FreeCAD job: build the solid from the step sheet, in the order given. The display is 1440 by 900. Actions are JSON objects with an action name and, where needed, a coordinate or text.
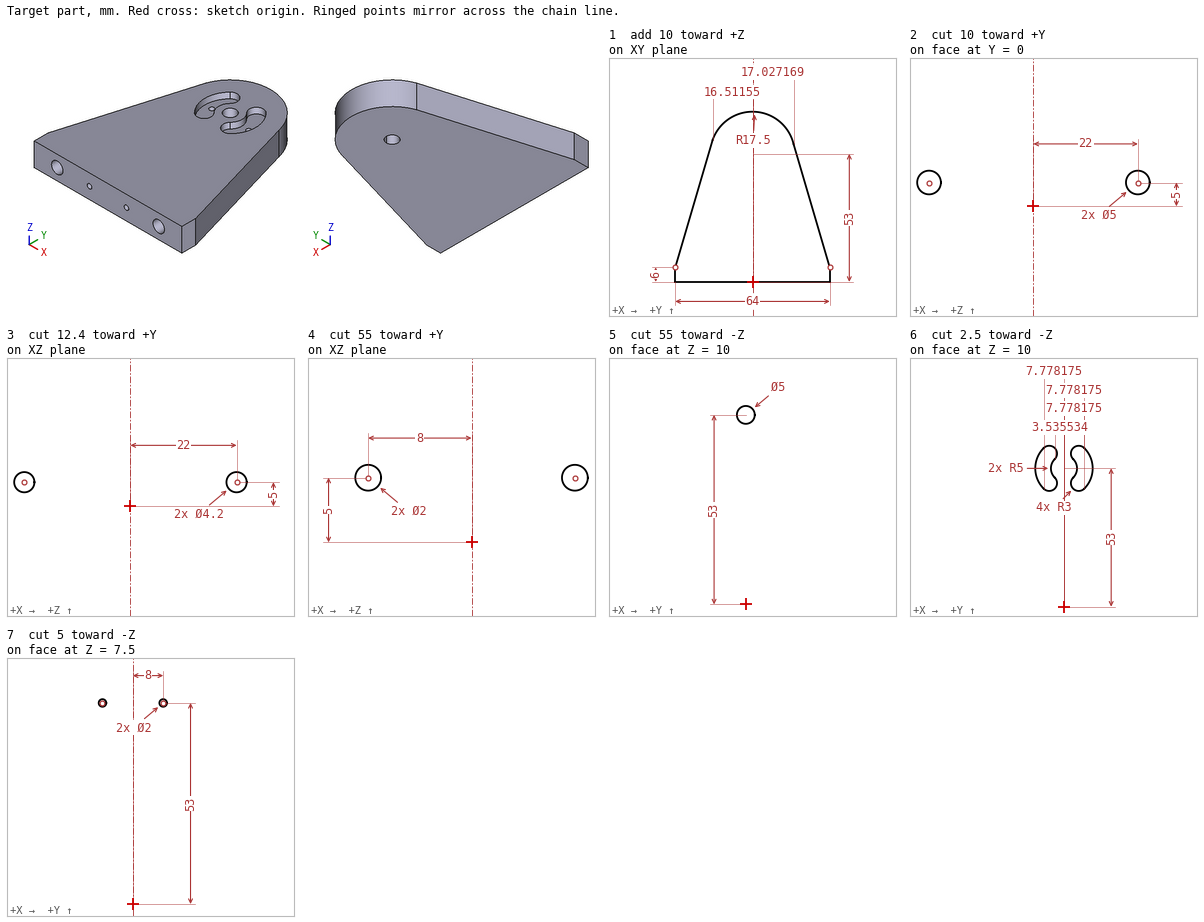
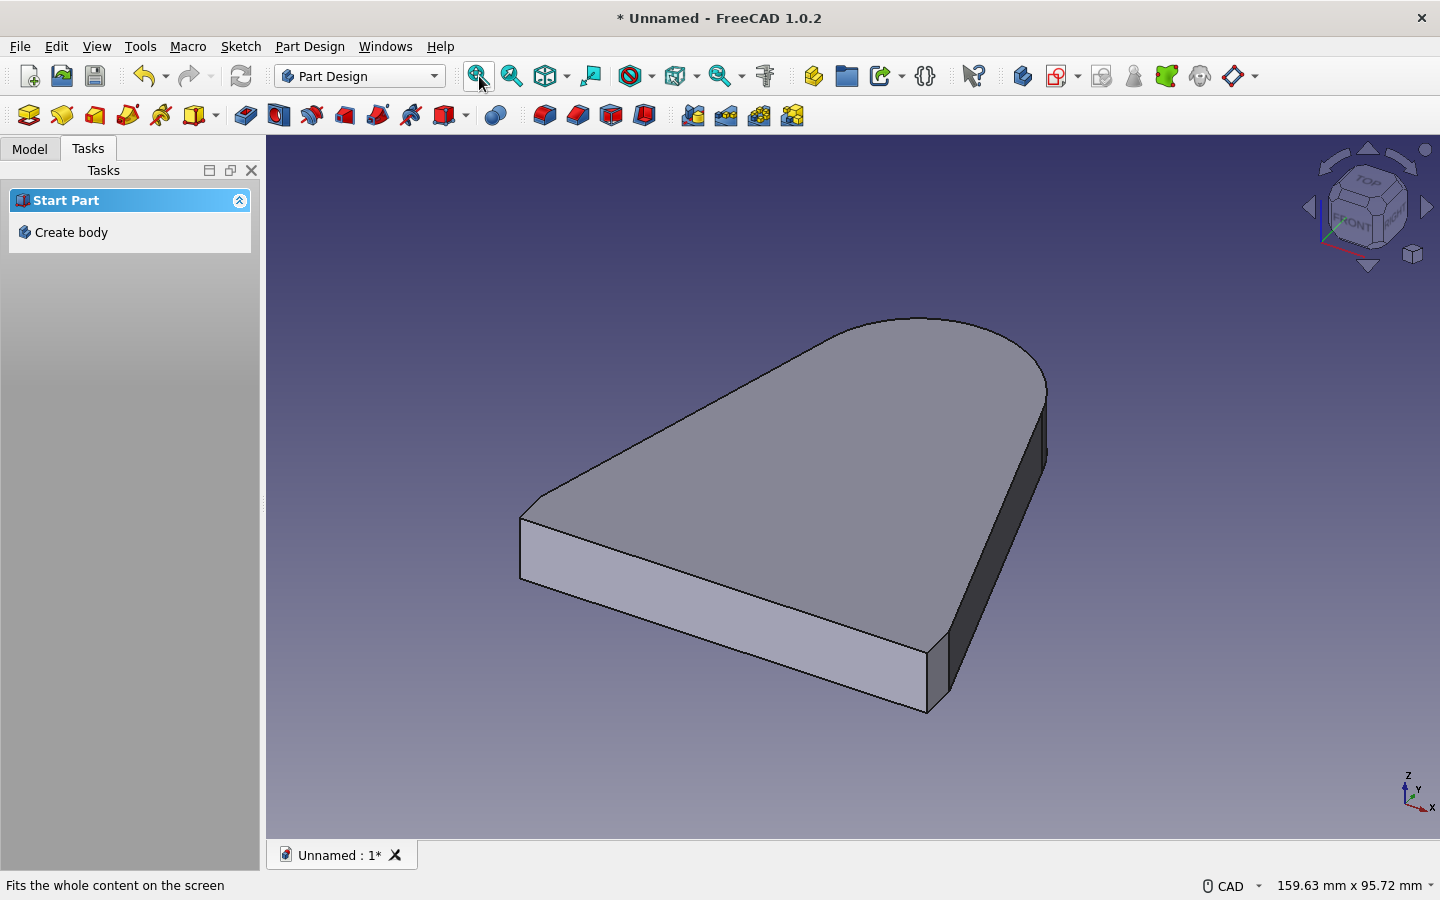
{"action": "left_click", "coordinate": [840, 653]}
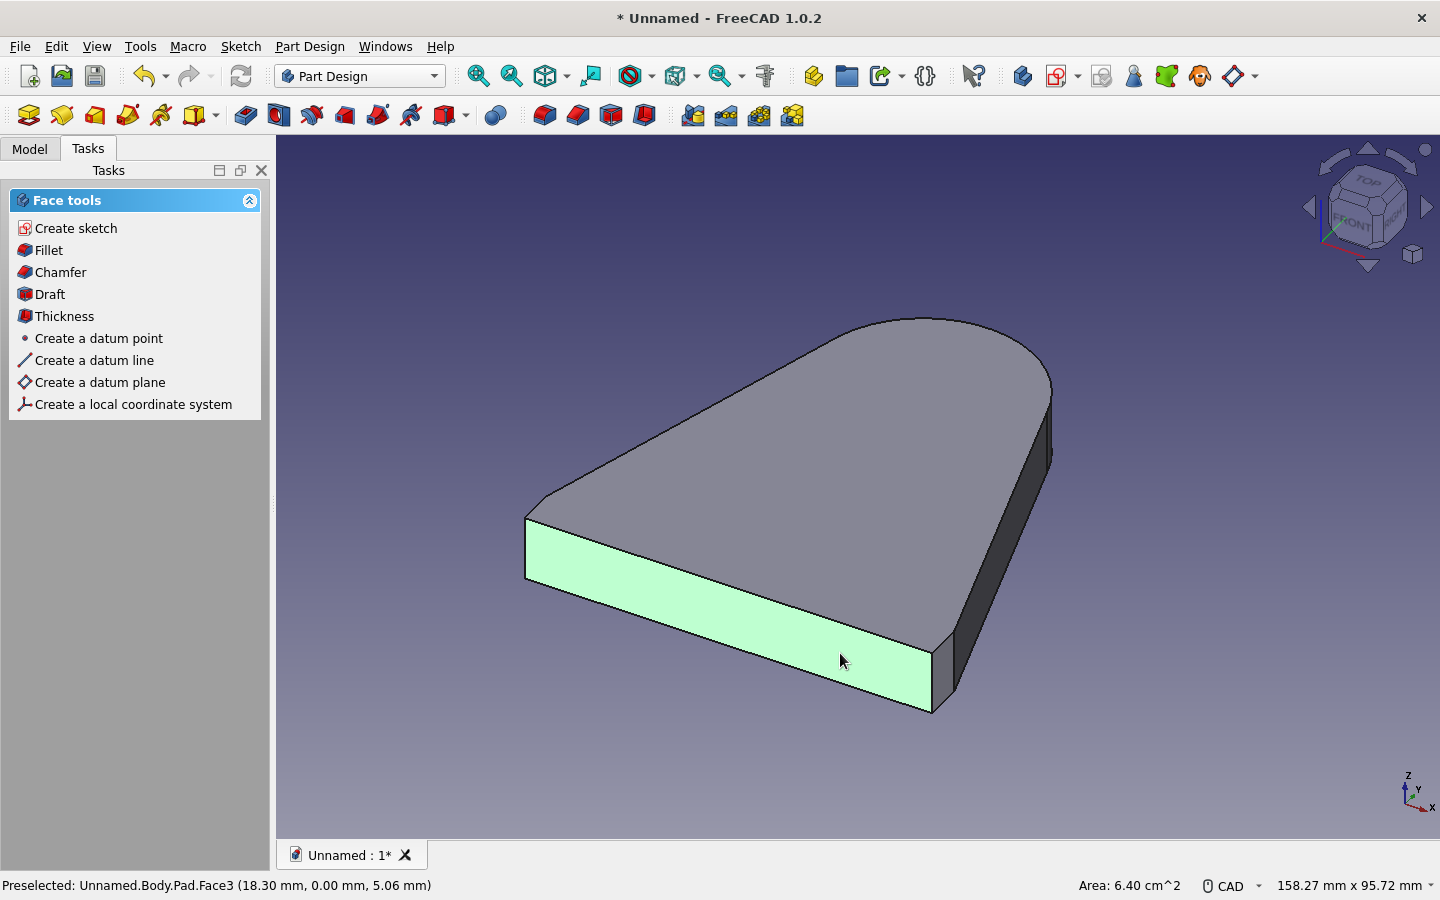
{"action": "left_click", "coordinate": [1056, 76]}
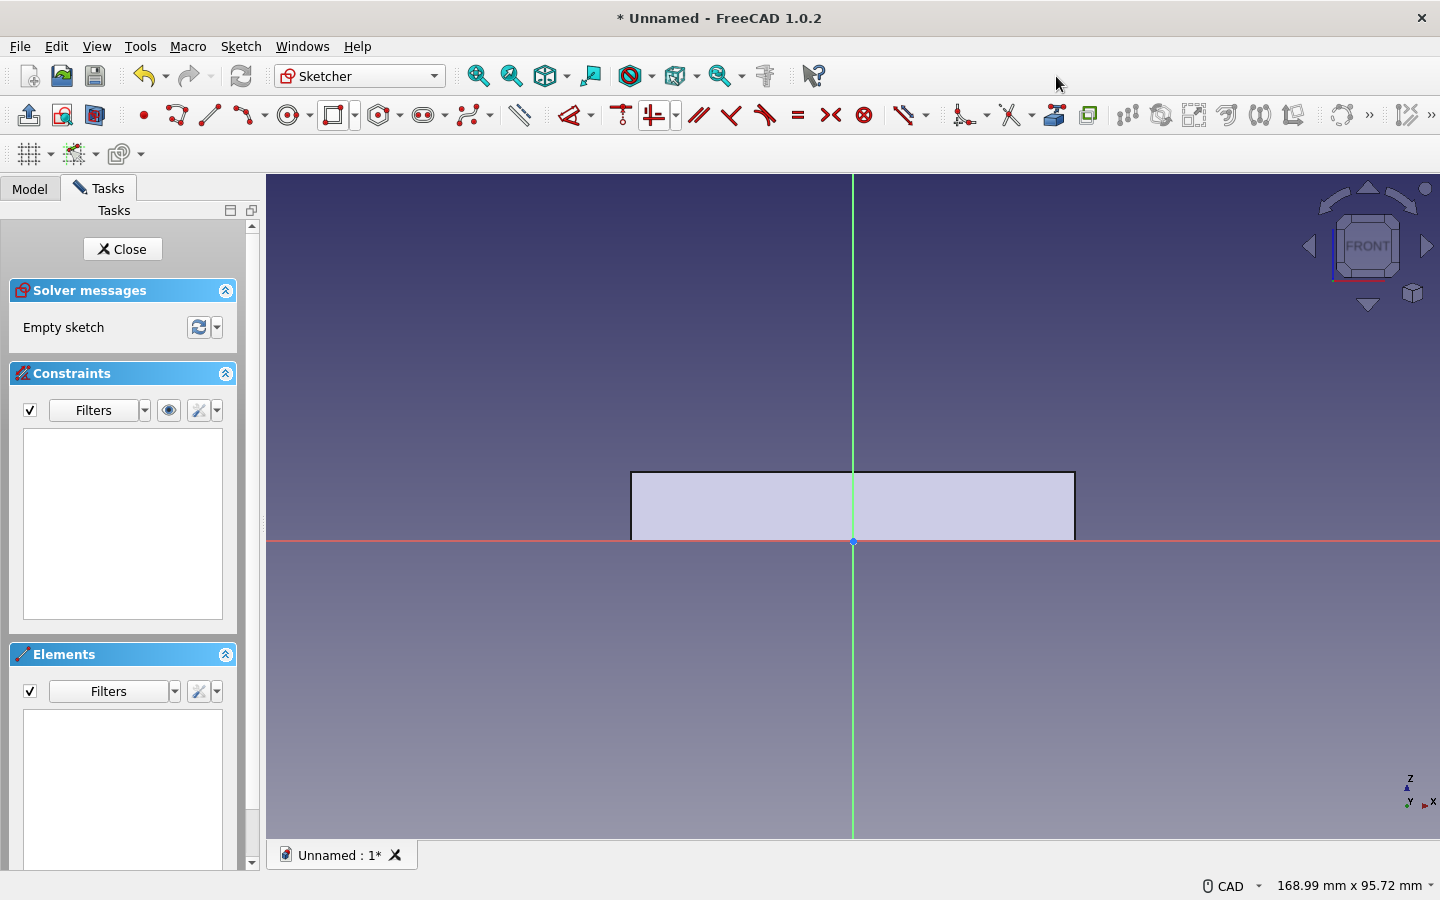
{"action": "scroll", "coordinate": [909, 522], "scroll_direction": "up", "scroll_amount": 4}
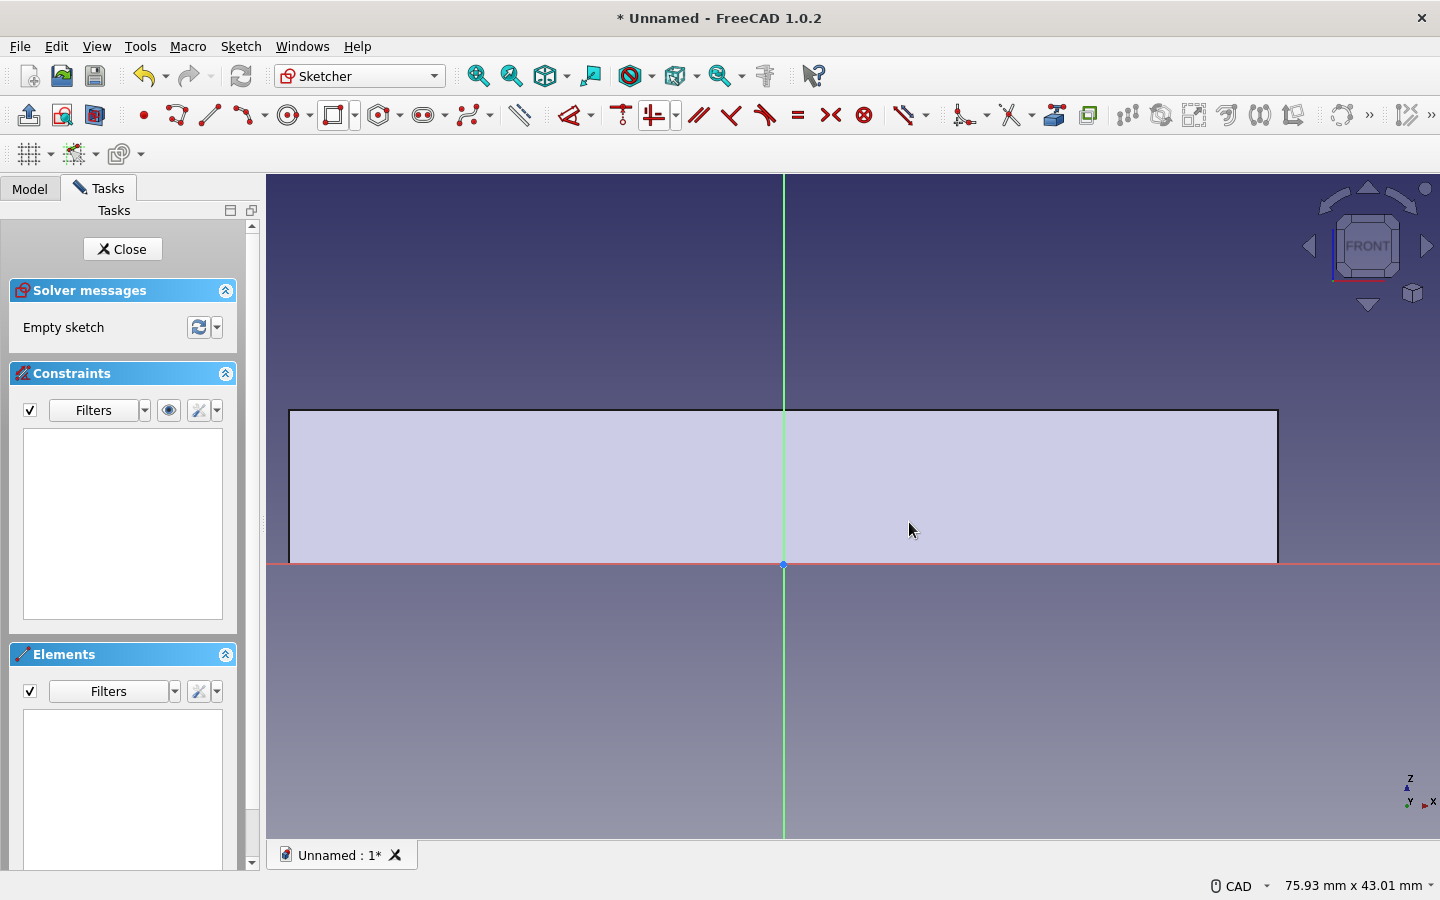
{"action": "left_click", "coordinate": [288, 116]}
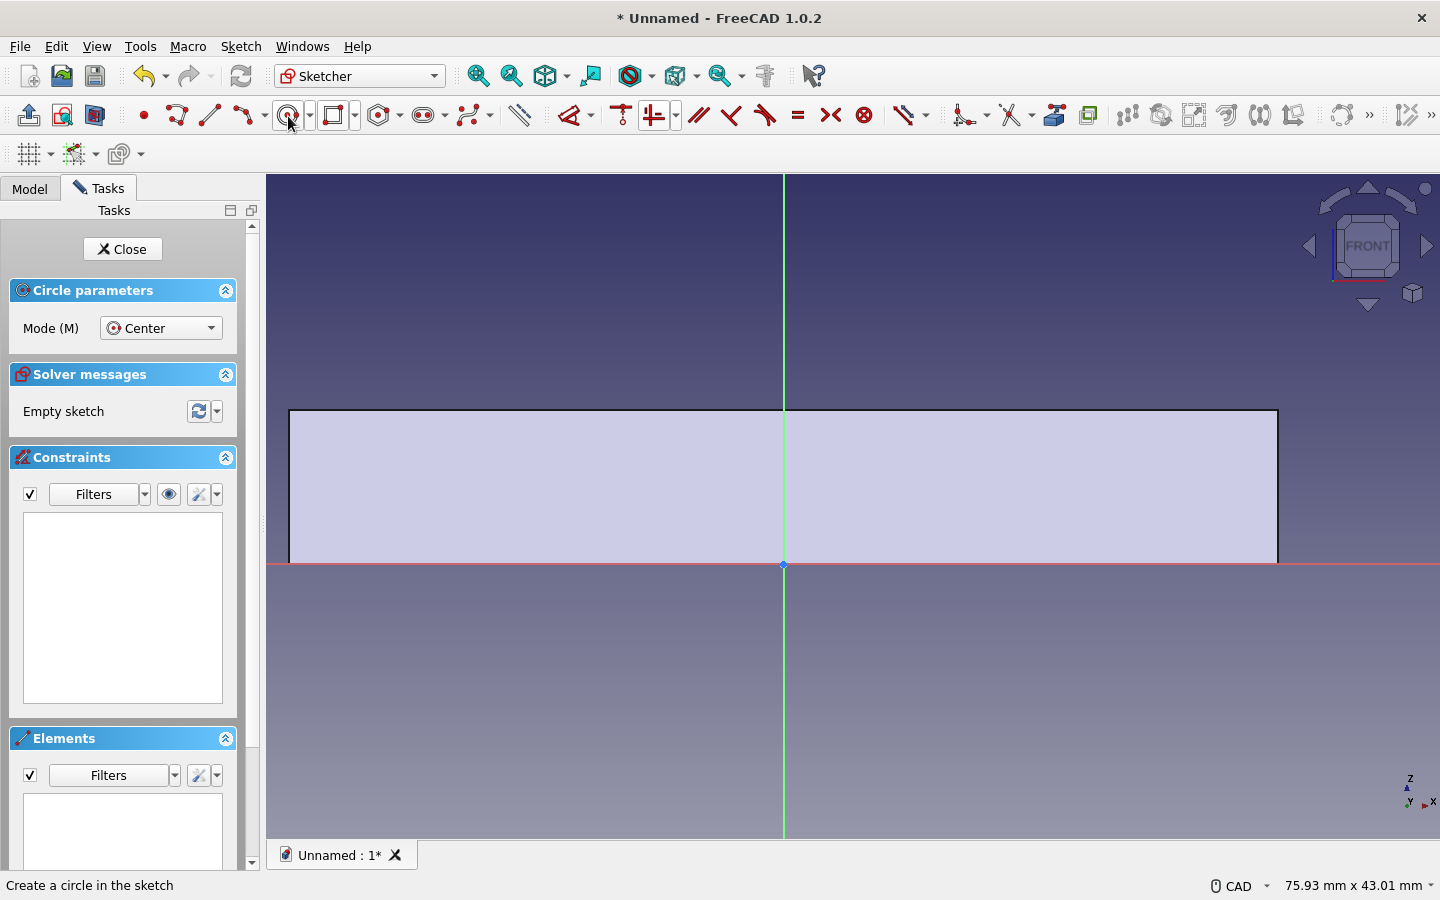
{"action": "left_click", "coordinate": [1124, 487]}
{"action": "mouse_move", "coordinate": [1151, 460]}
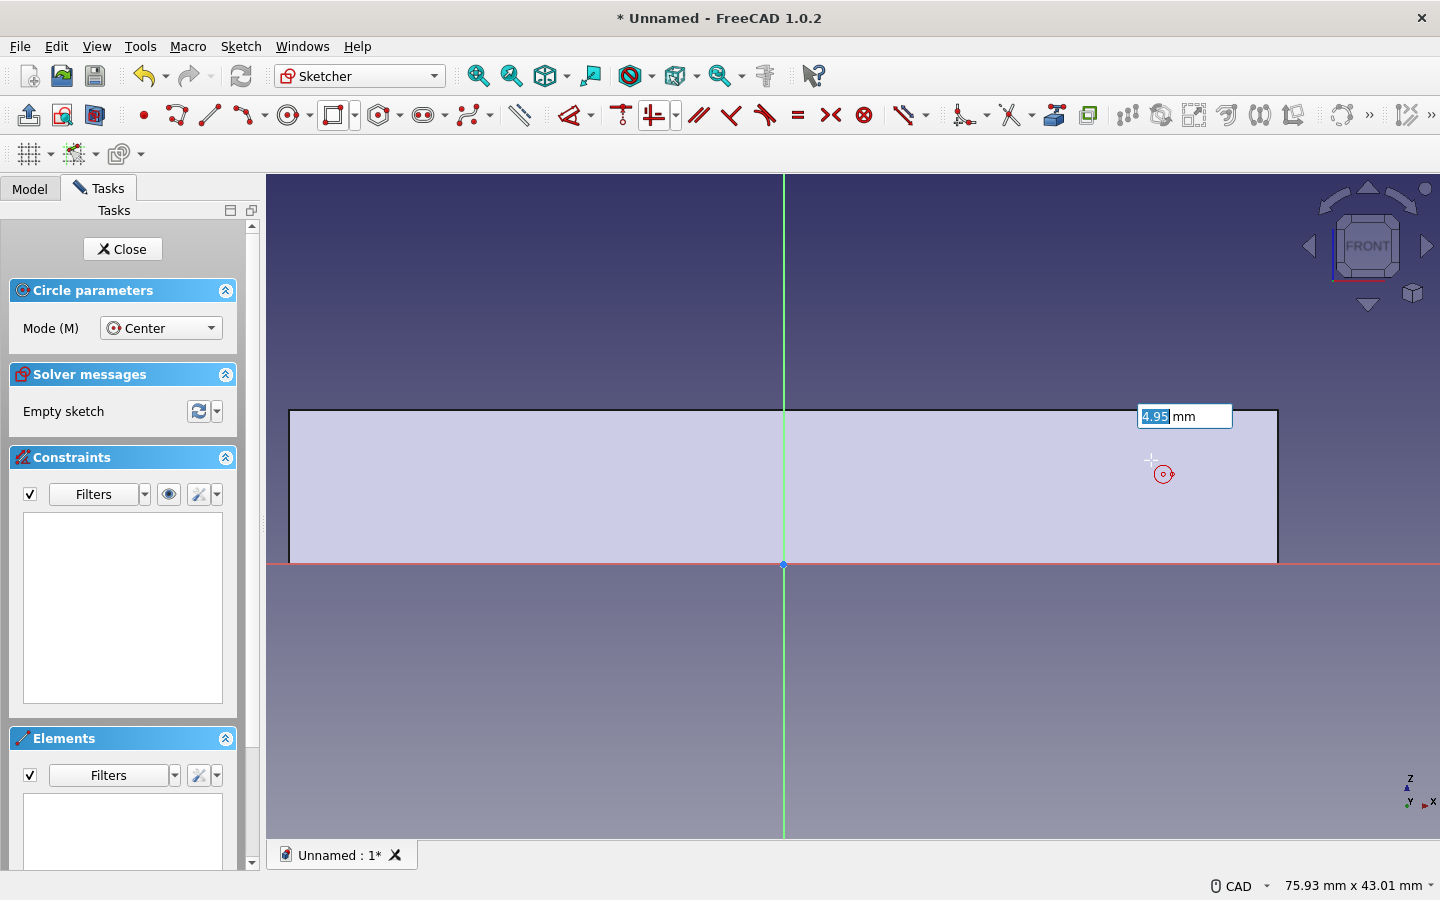
{"action": "type", "text": "5"}
{"action": "key", "text": "Return"}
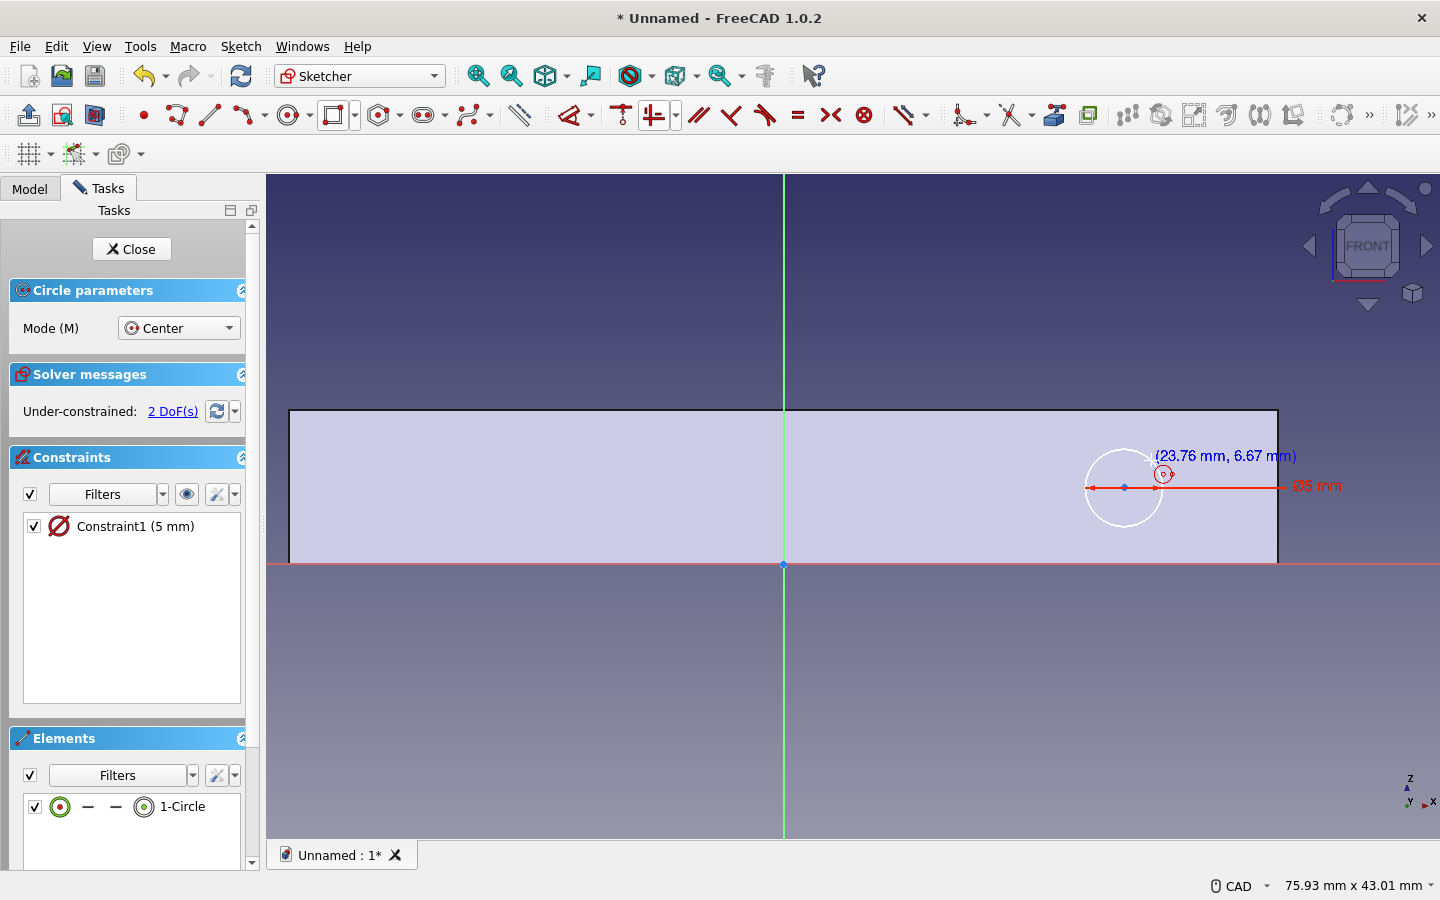
{"action": "left_click", "coordinate": [444, 487]}
{"action": "mouse_move", "coordinate": [471, 460]}